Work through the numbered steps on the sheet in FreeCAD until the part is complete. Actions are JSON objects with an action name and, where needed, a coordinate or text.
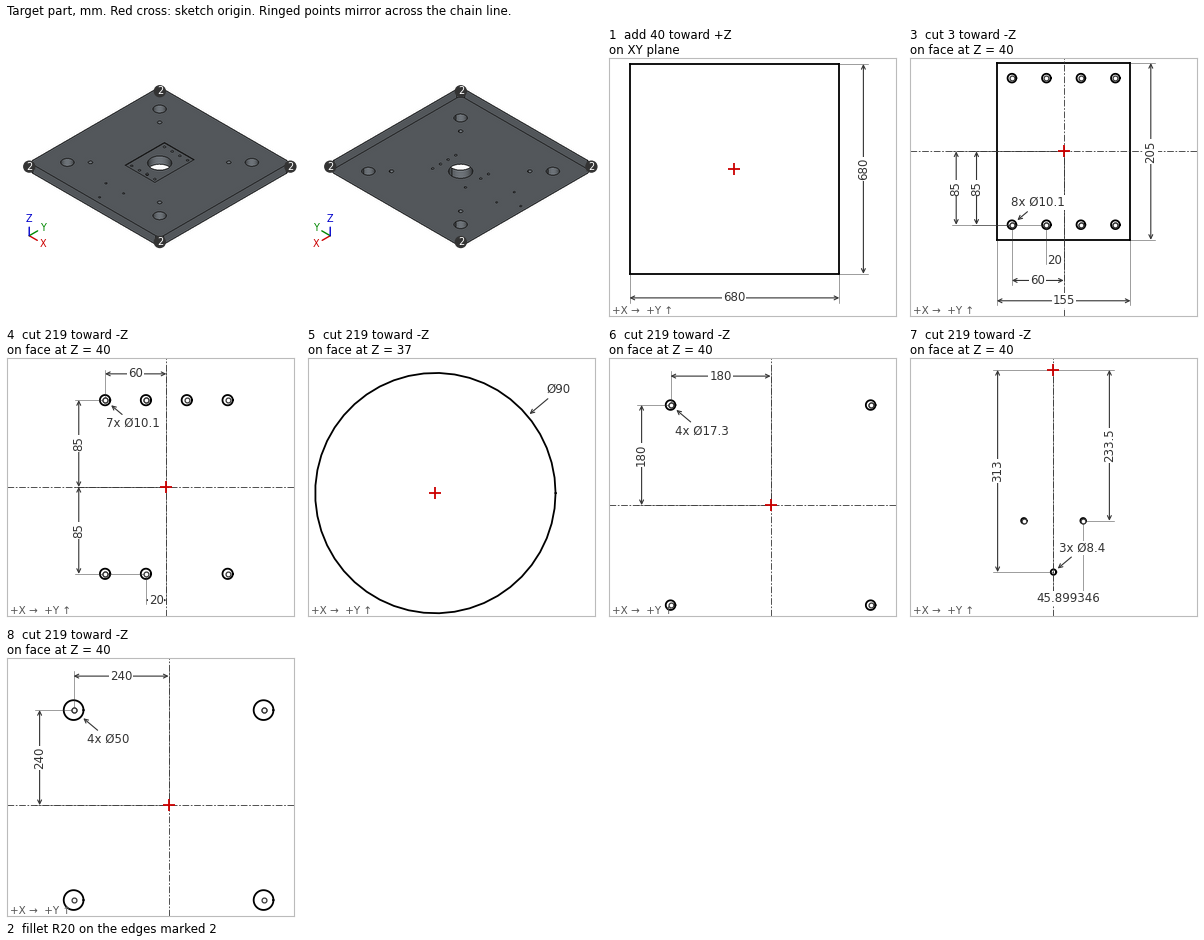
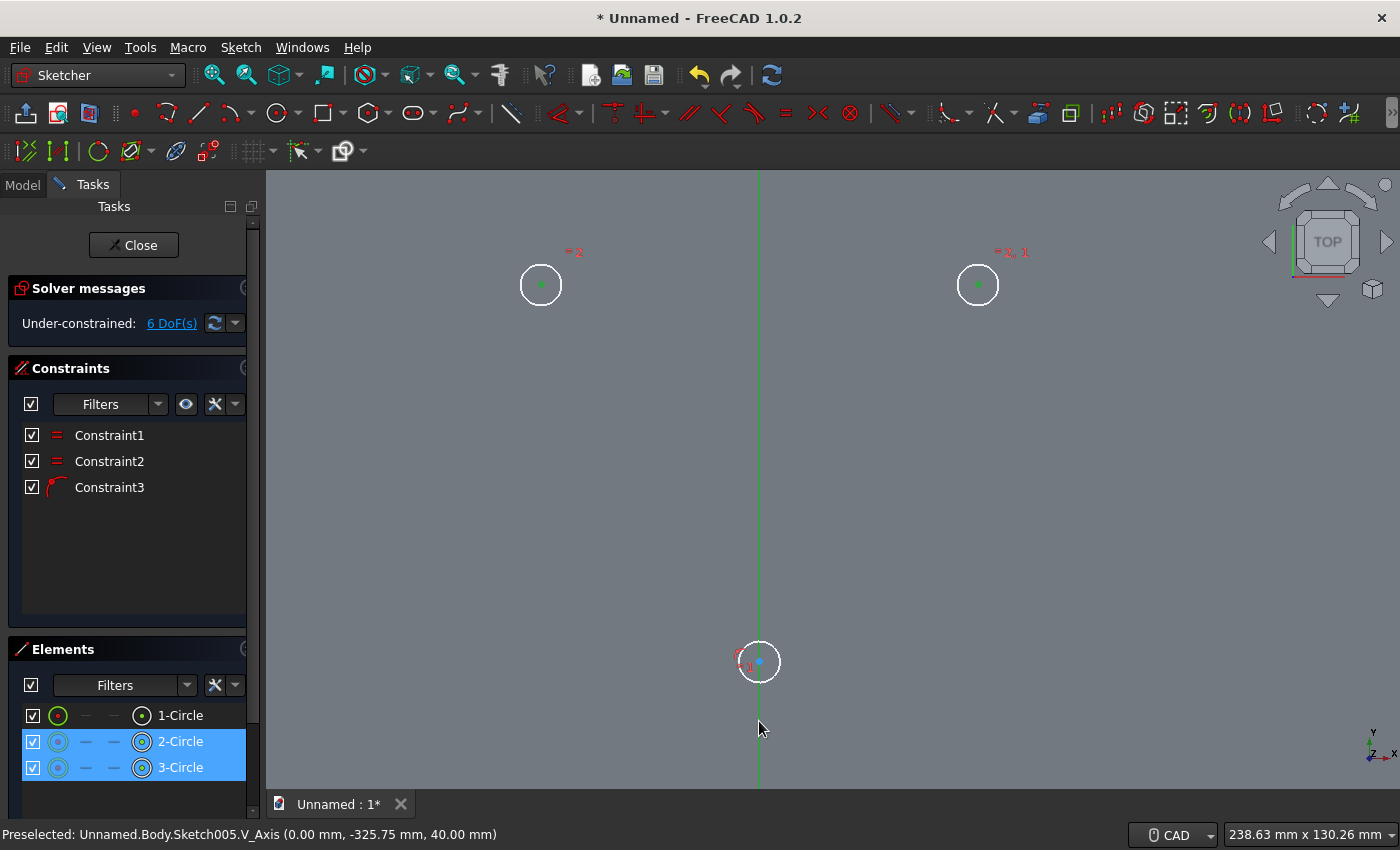
{"action": "left_click", "coordinate": [818, 114]}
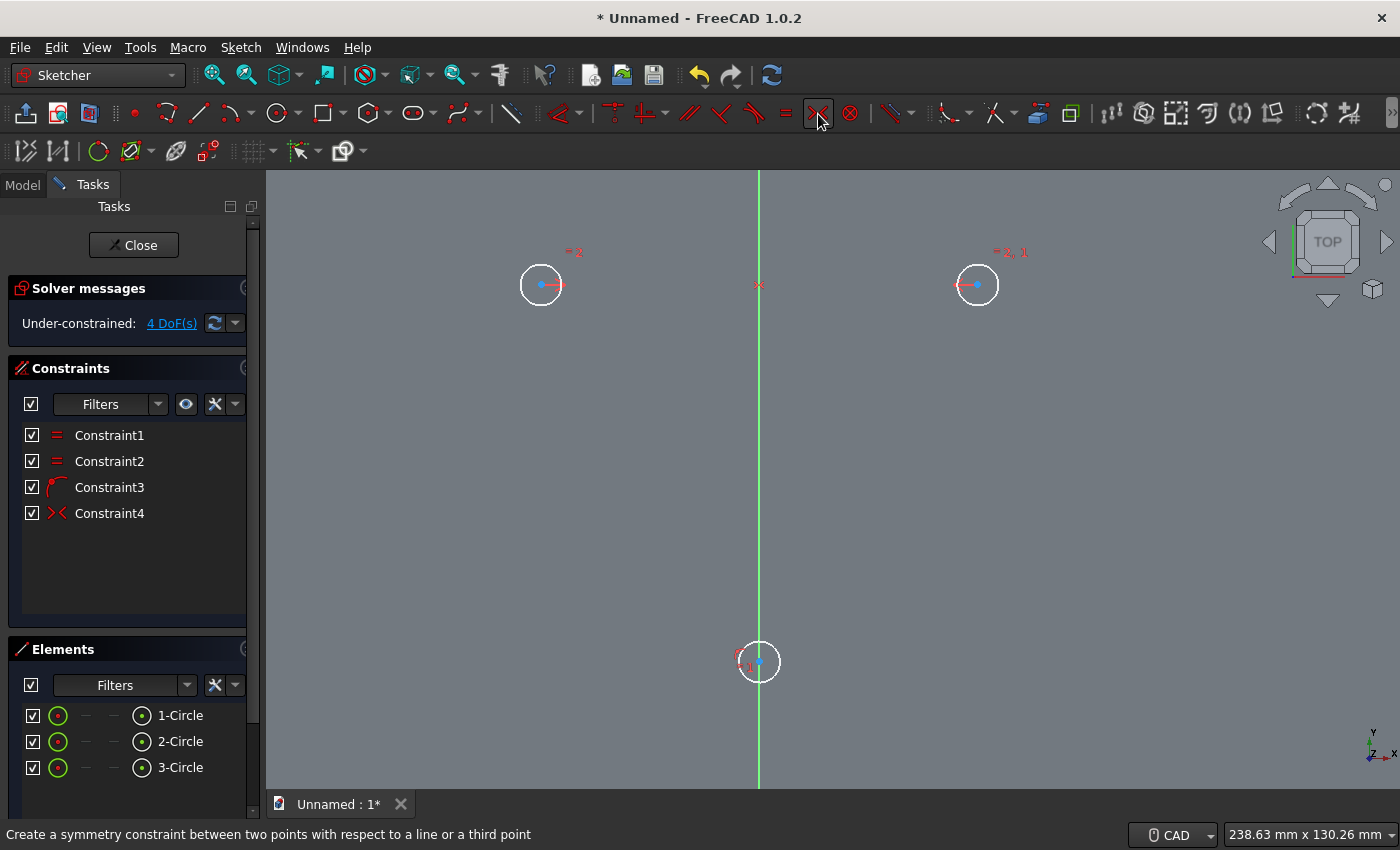
{"action": "left_click", "coordinate": [558, 114]}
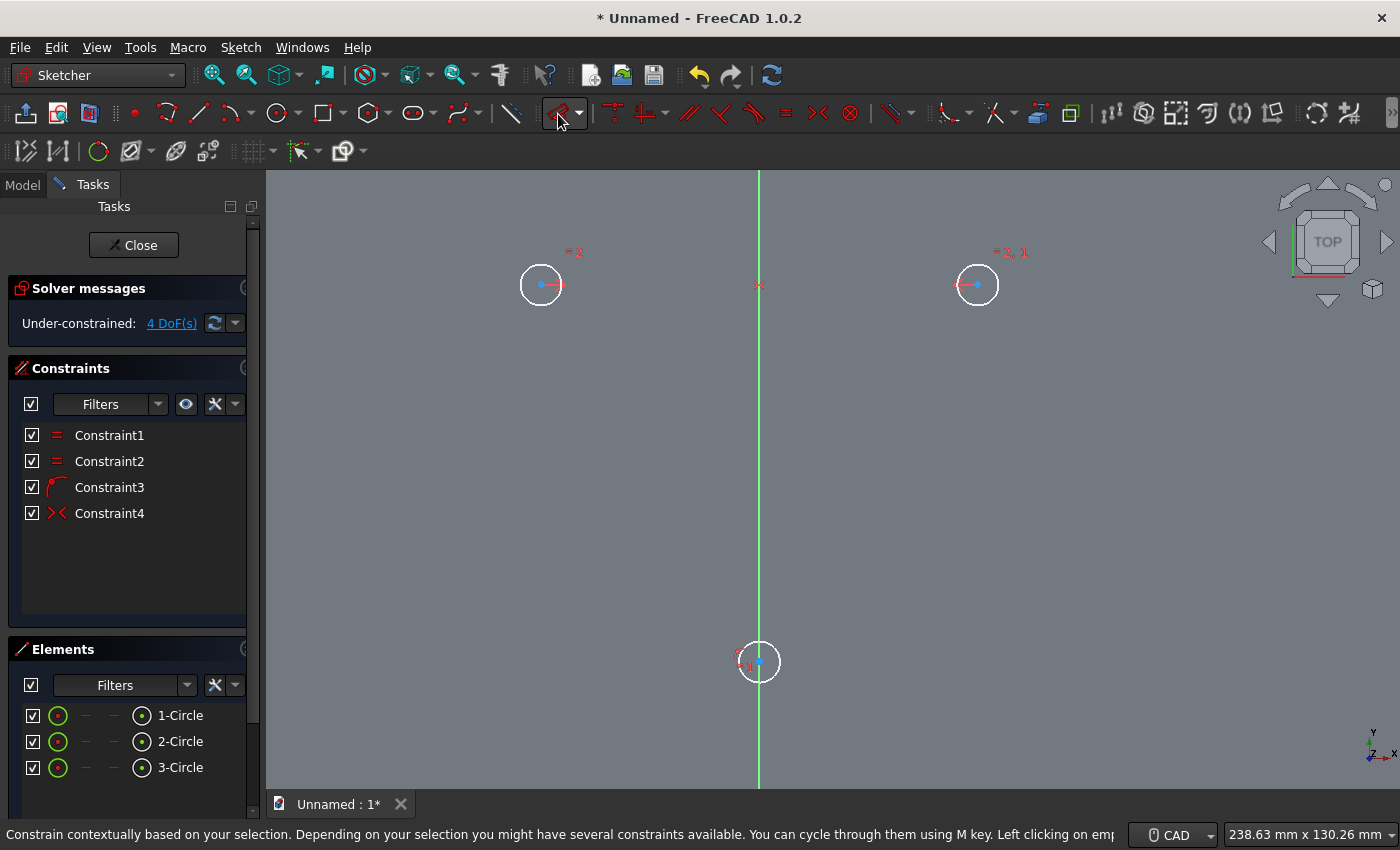
{"action": "left_click", "coordinate": [774, 647]}
{"action": "left_click", "coordinate": [796, 624]}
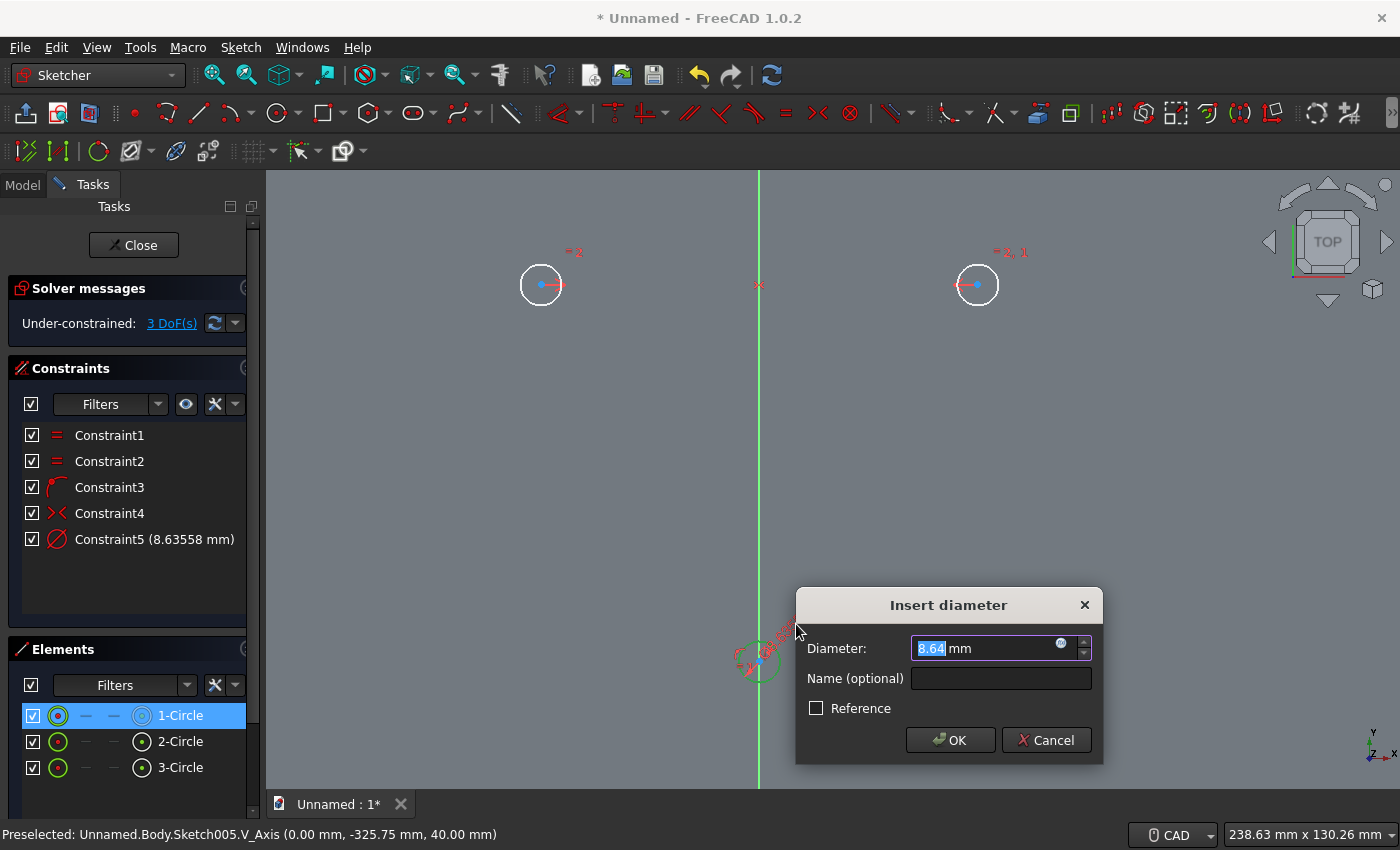
{"action": "type", "text": "8.4"}
{"action": "key", "text": "Return"}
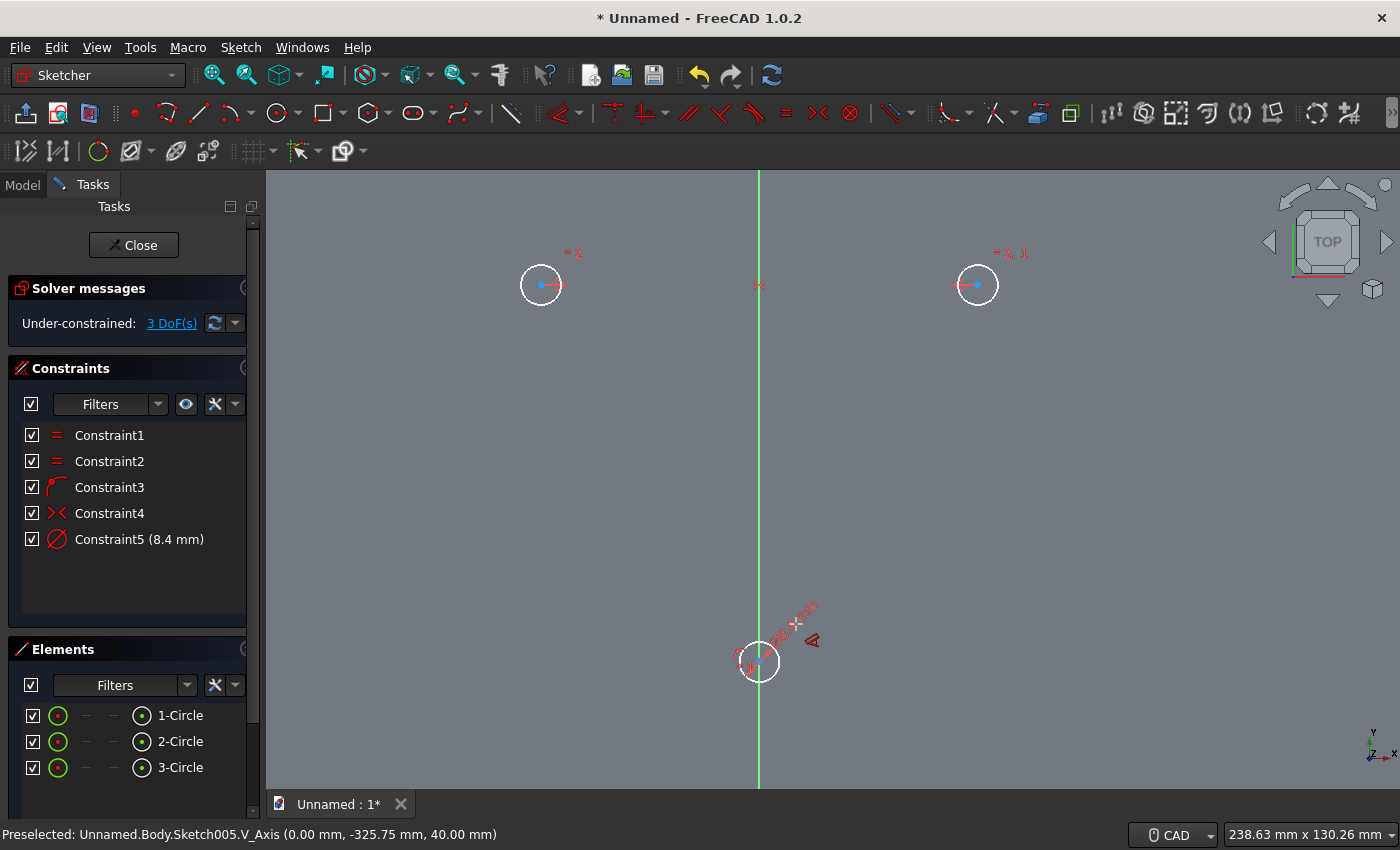
{"action": "left_click", "coordinate": [759, 662]}
{"action": "left_click", "coordinate": [793, 430]}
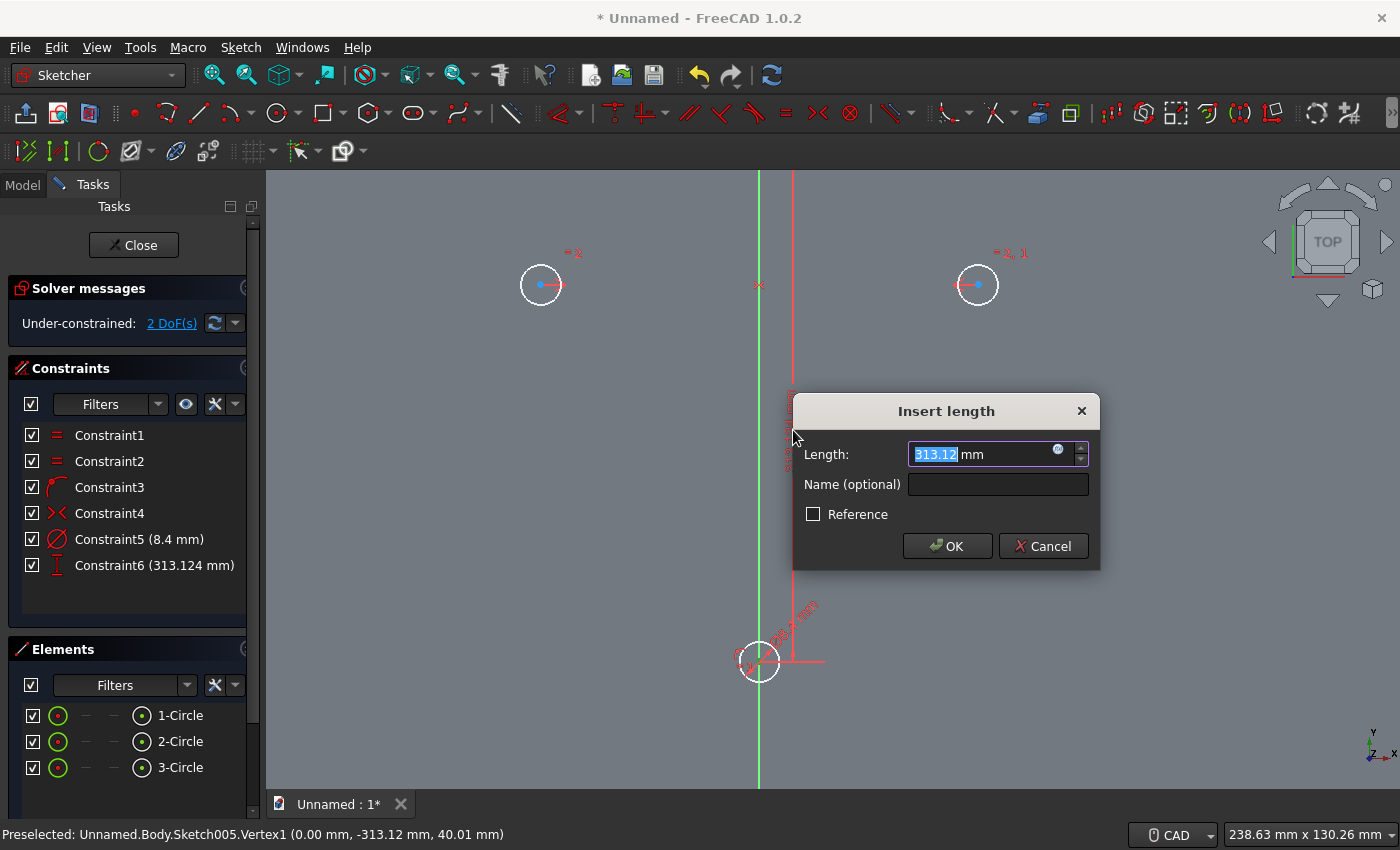
{"action": "type", "text": "313"}
{"action": "key", "text": "Return"}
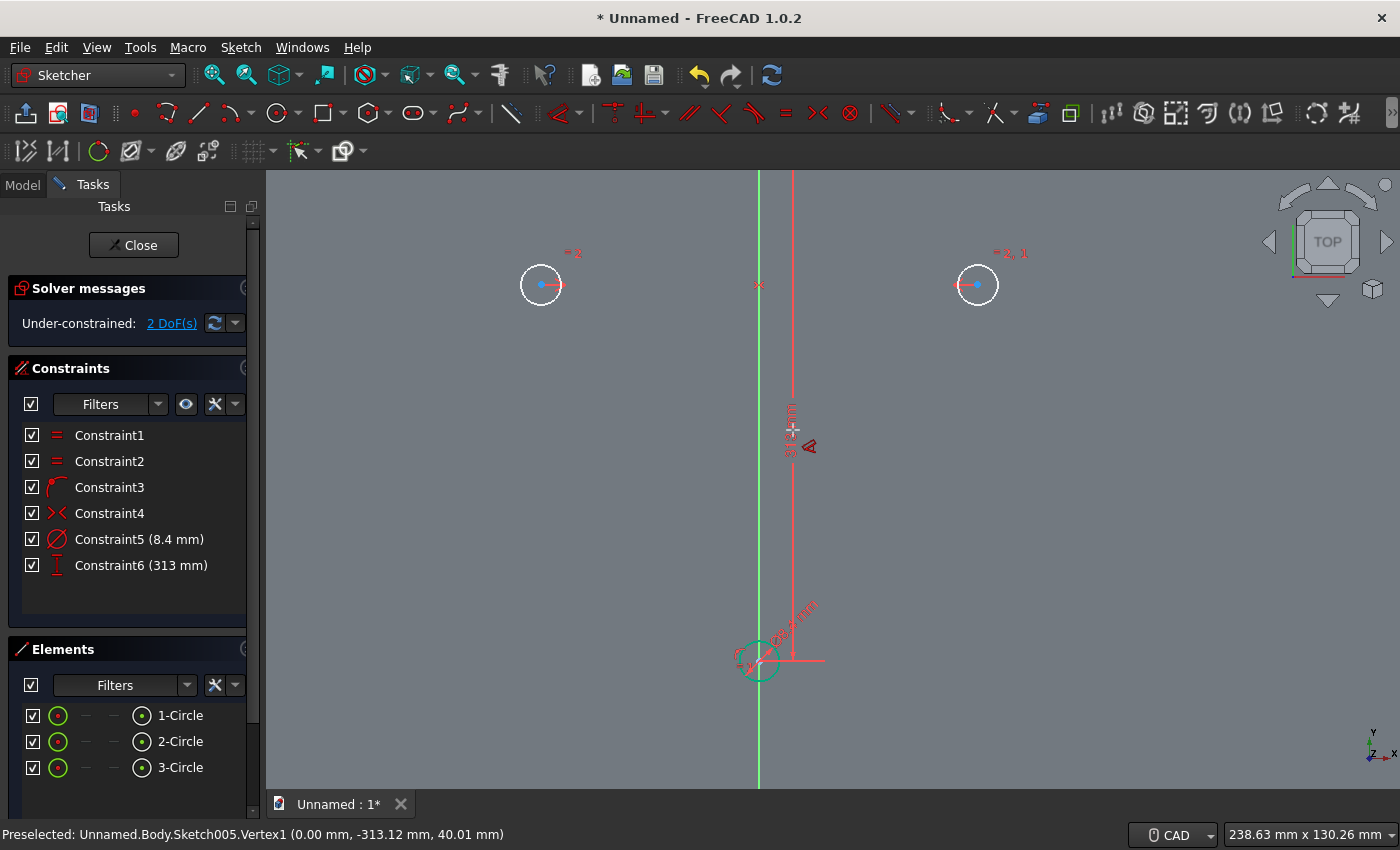
{"action": "left_click", "coordinate": [978, 285]}
{"action": "left_click", "coordinate": [1012, 242]}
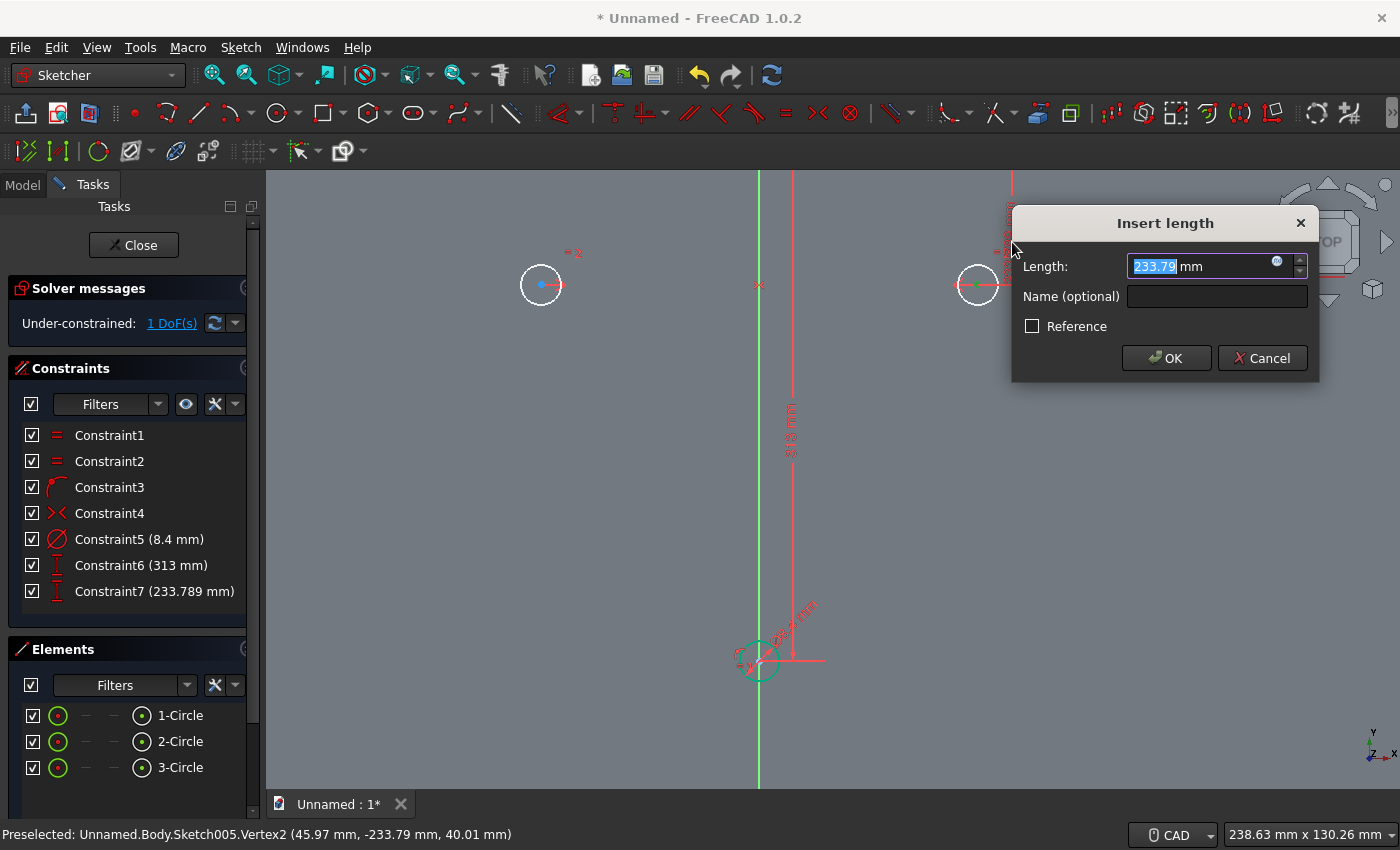
{"action": "type", "text": "233.5"}
{"action": "key", "text": "Return"}